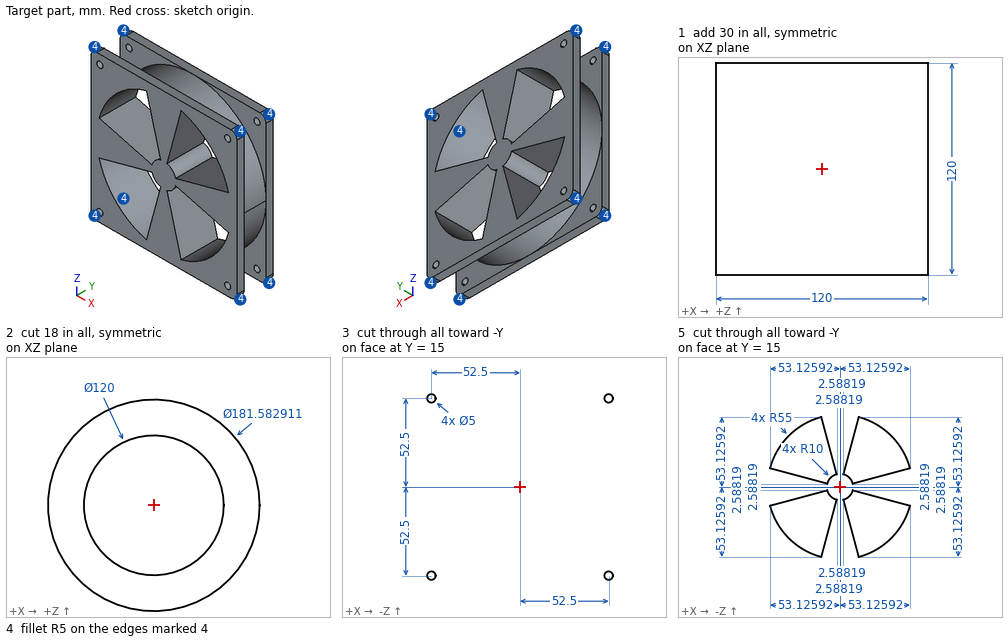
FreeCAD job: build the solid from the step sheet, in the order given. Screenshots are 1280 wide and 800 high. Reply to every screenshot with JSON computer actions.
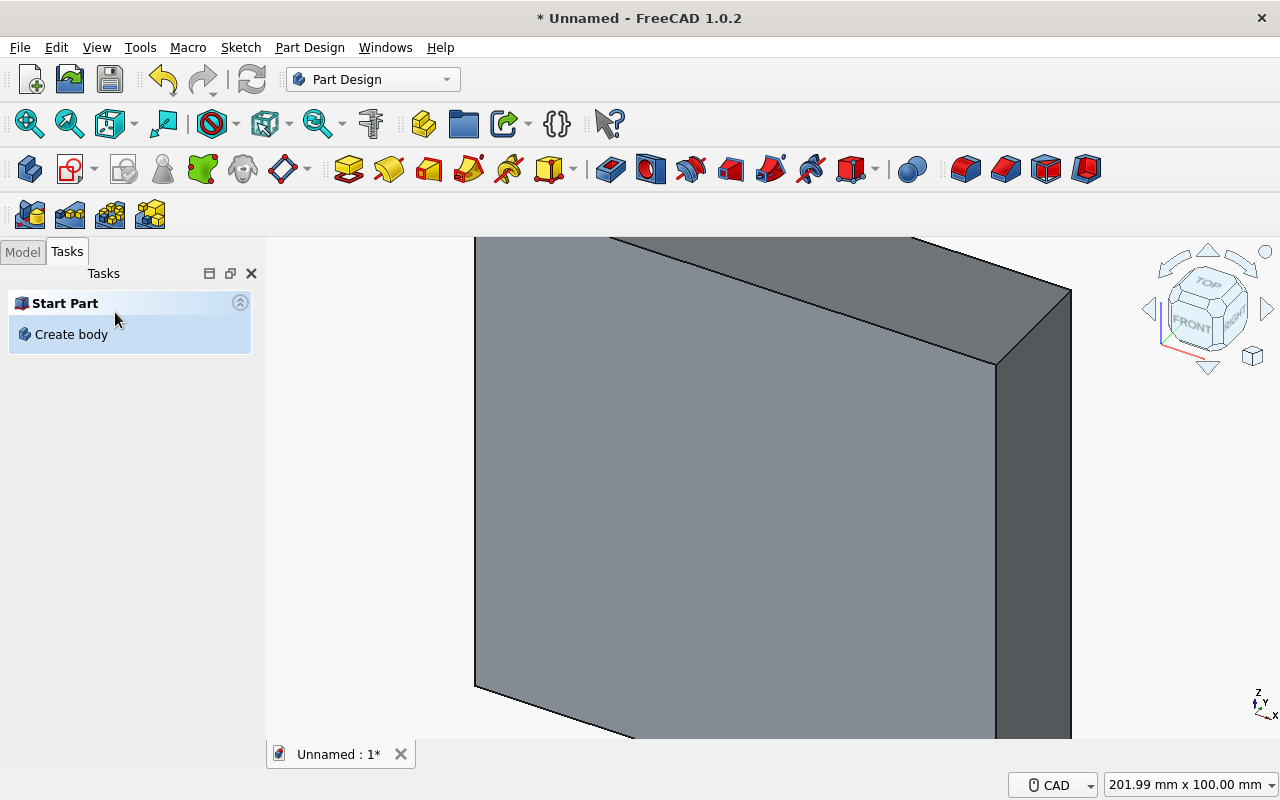
{"action": "left_click", "coordinate": [30, 124]}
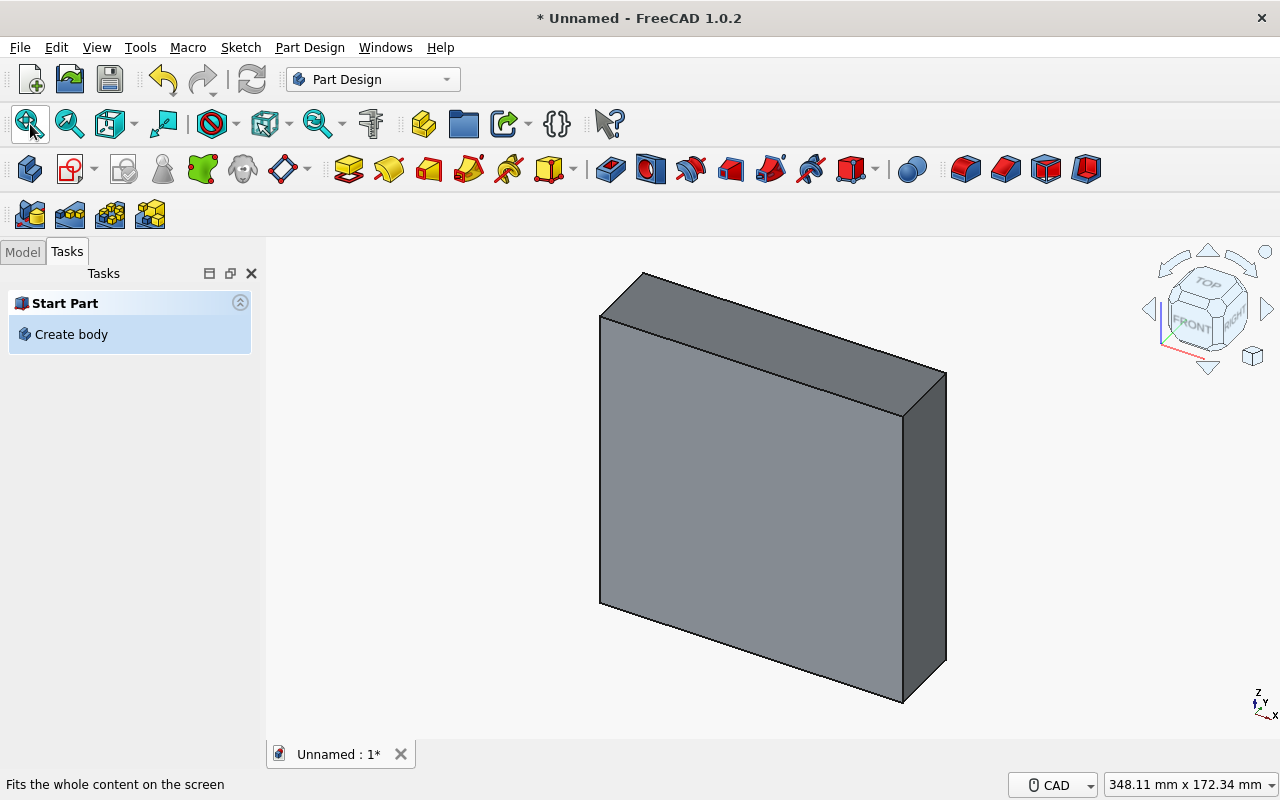
{"action": "left_click", "coordinate": [70, 170]}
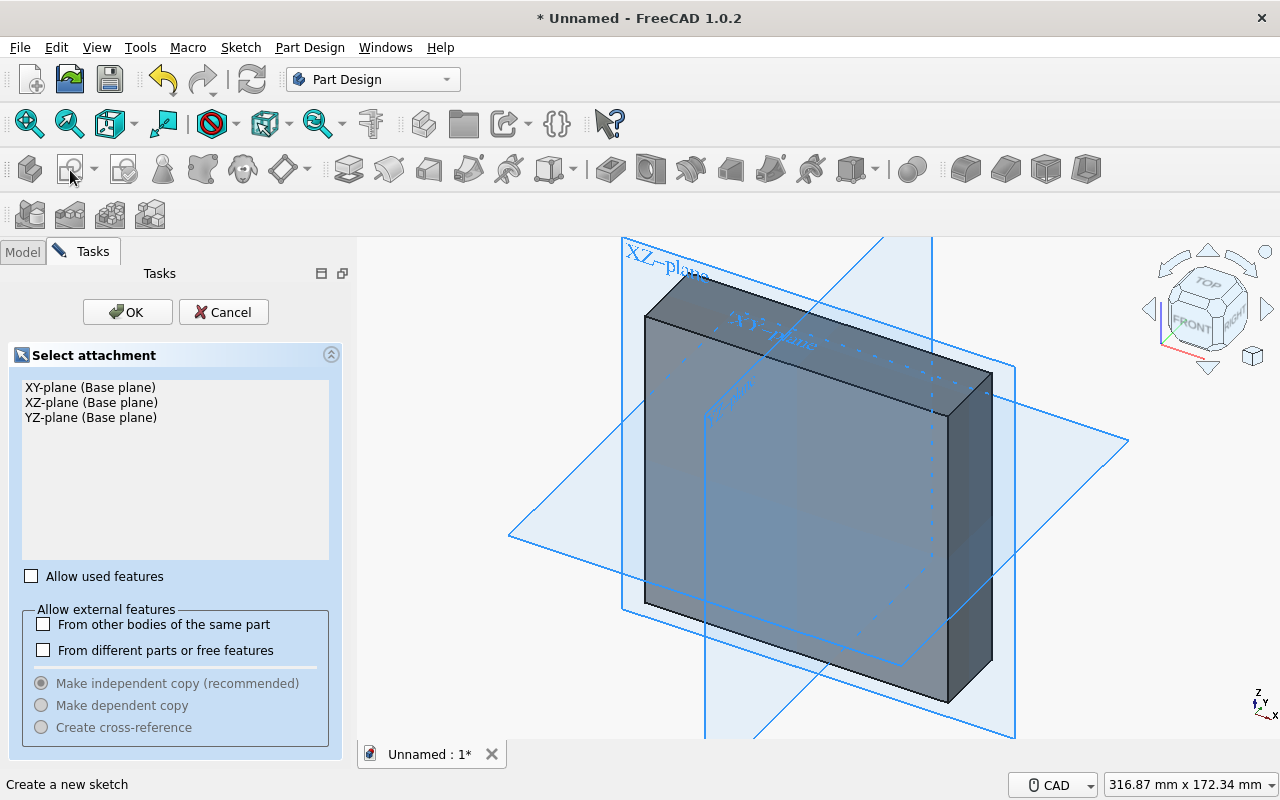
{"action": "left_click", "coordinate": [82, 402]}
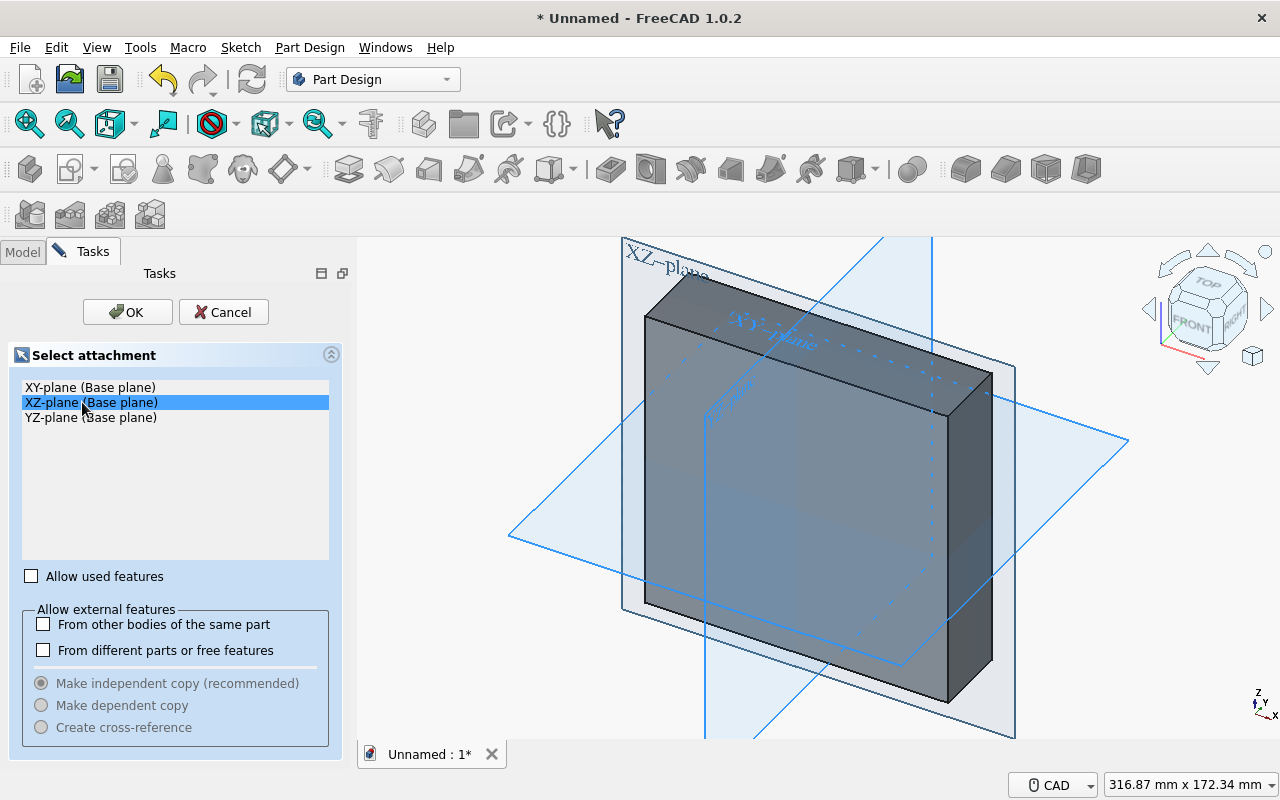
{"action": "left_click", "coordinate": [128, 312]}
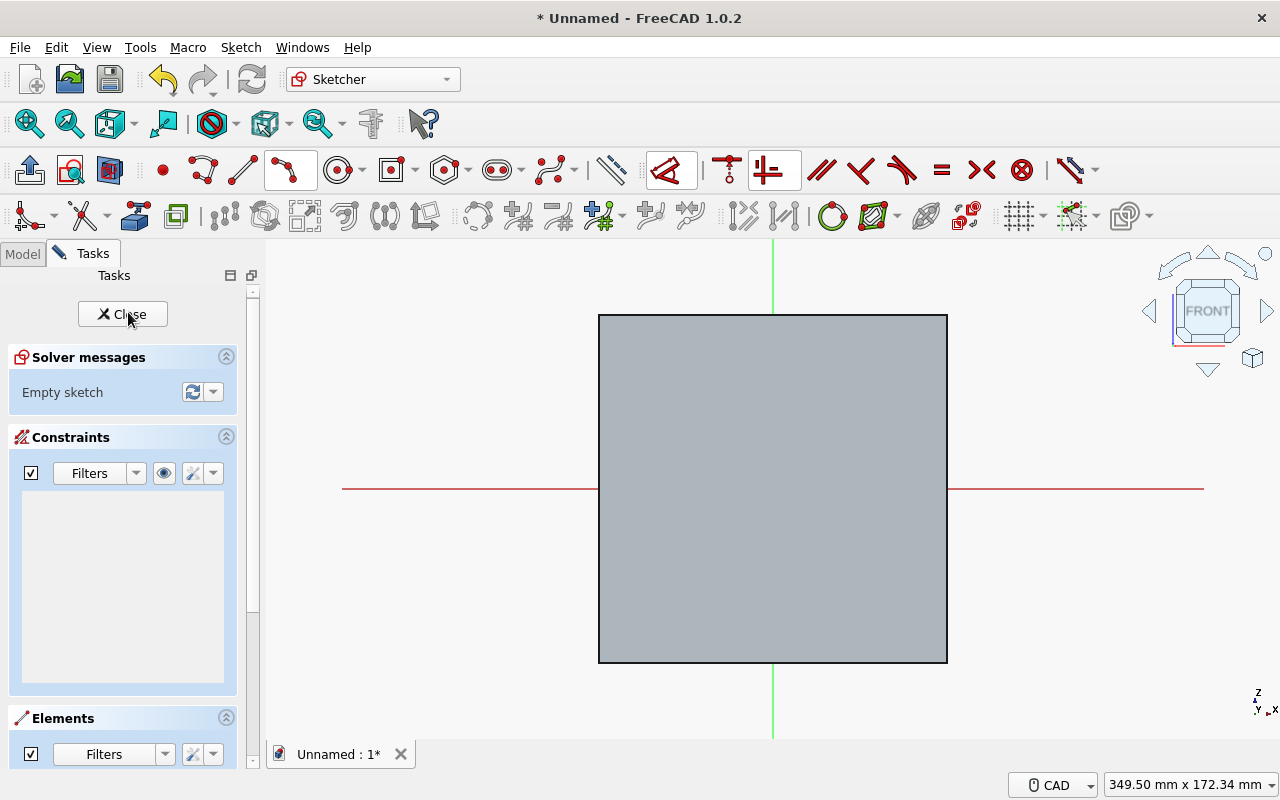
{"action": "left_click", "coordinate": [110, 170]}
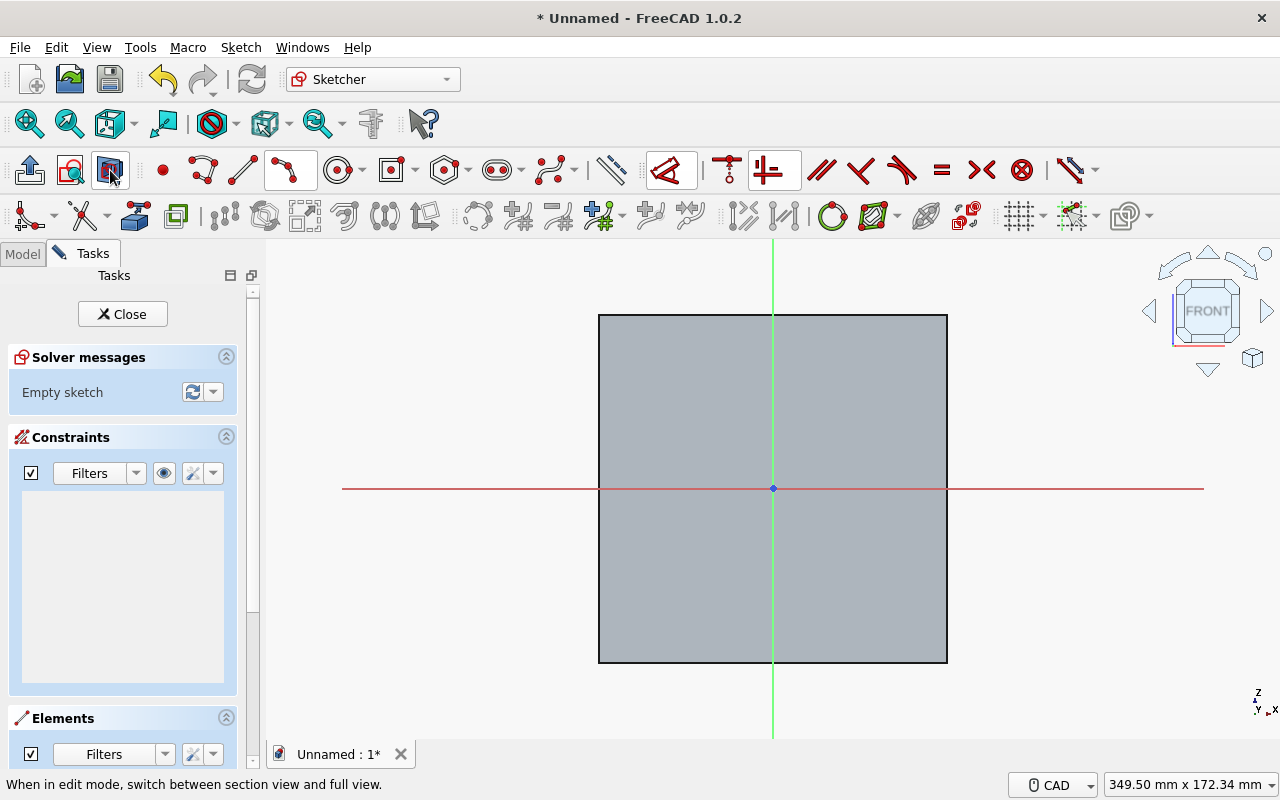
{"action": "scroll", "coordinate": [621, 489], "scroll_direction": "down", "scroll_amount": 3}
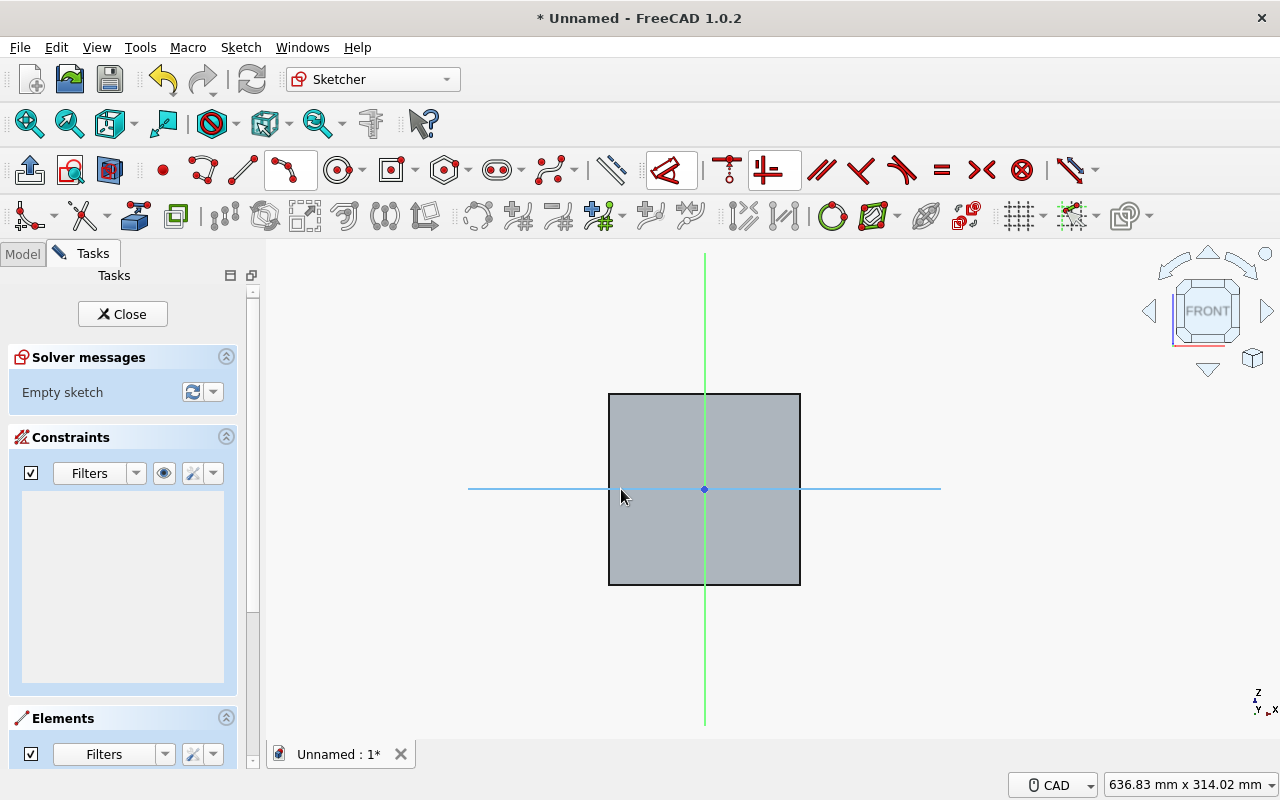
{"action": "left_click", "coordinate": [338, 170]}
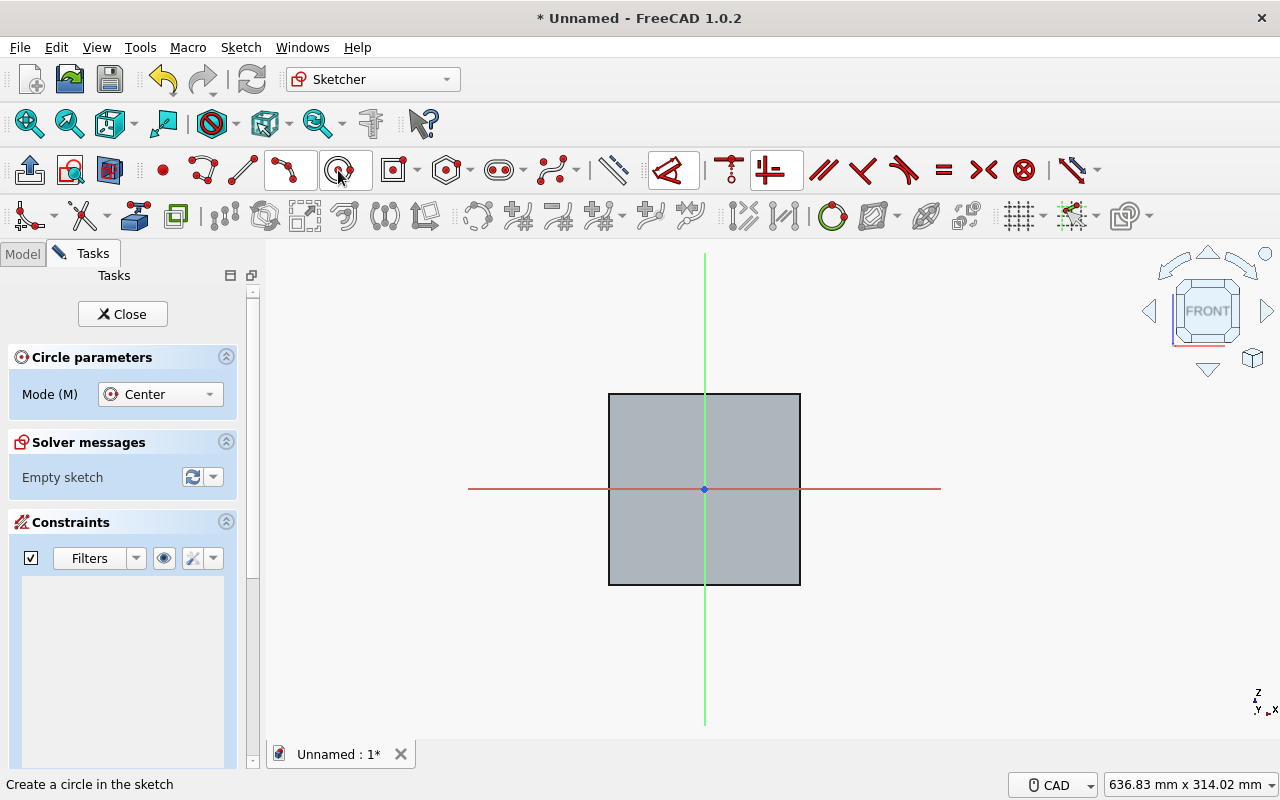
{"action": "left_click", "coordinate": [705, 489]}
{"action": "left_click", "coordinate": [807, 387]}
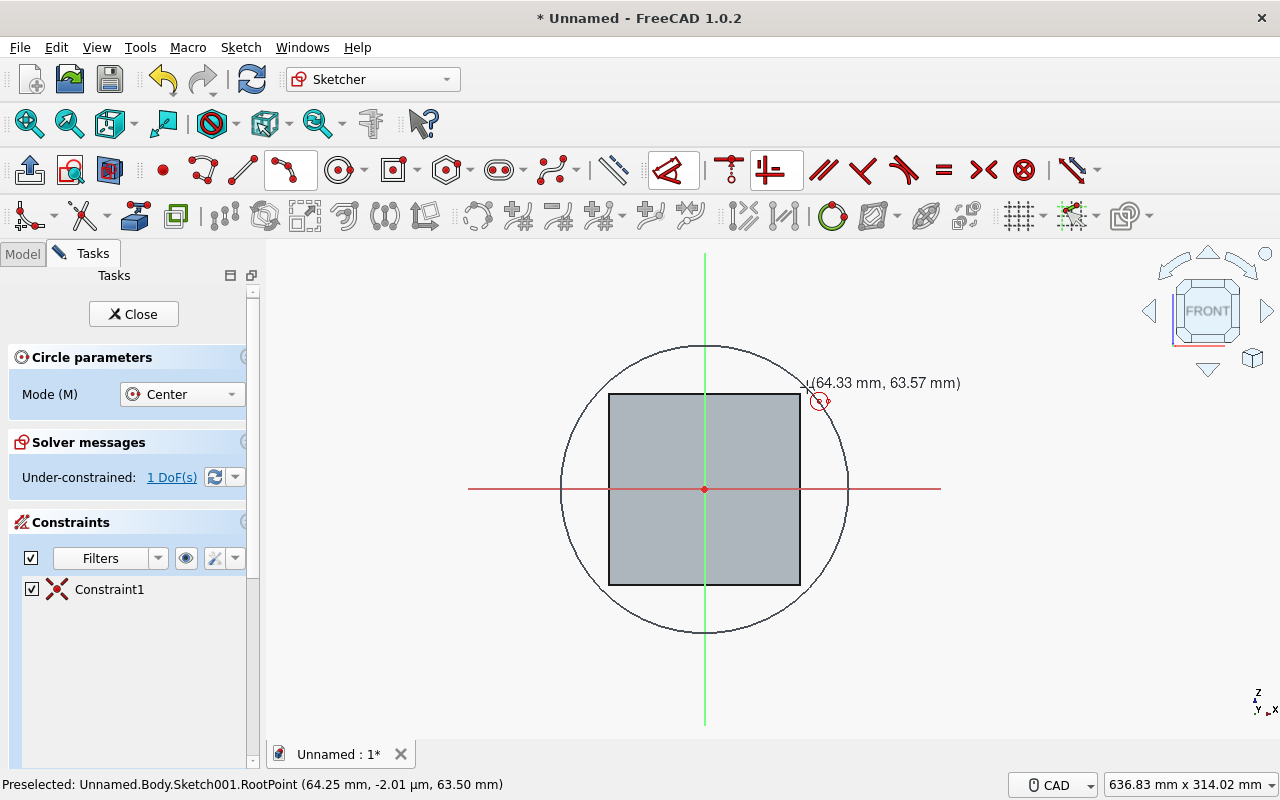
{"action": "left_click", "coordinate": [705, 489]}
{"action": "left_click", "coordinate": [772, 422]}
{"action": "key", "text": "Escape"}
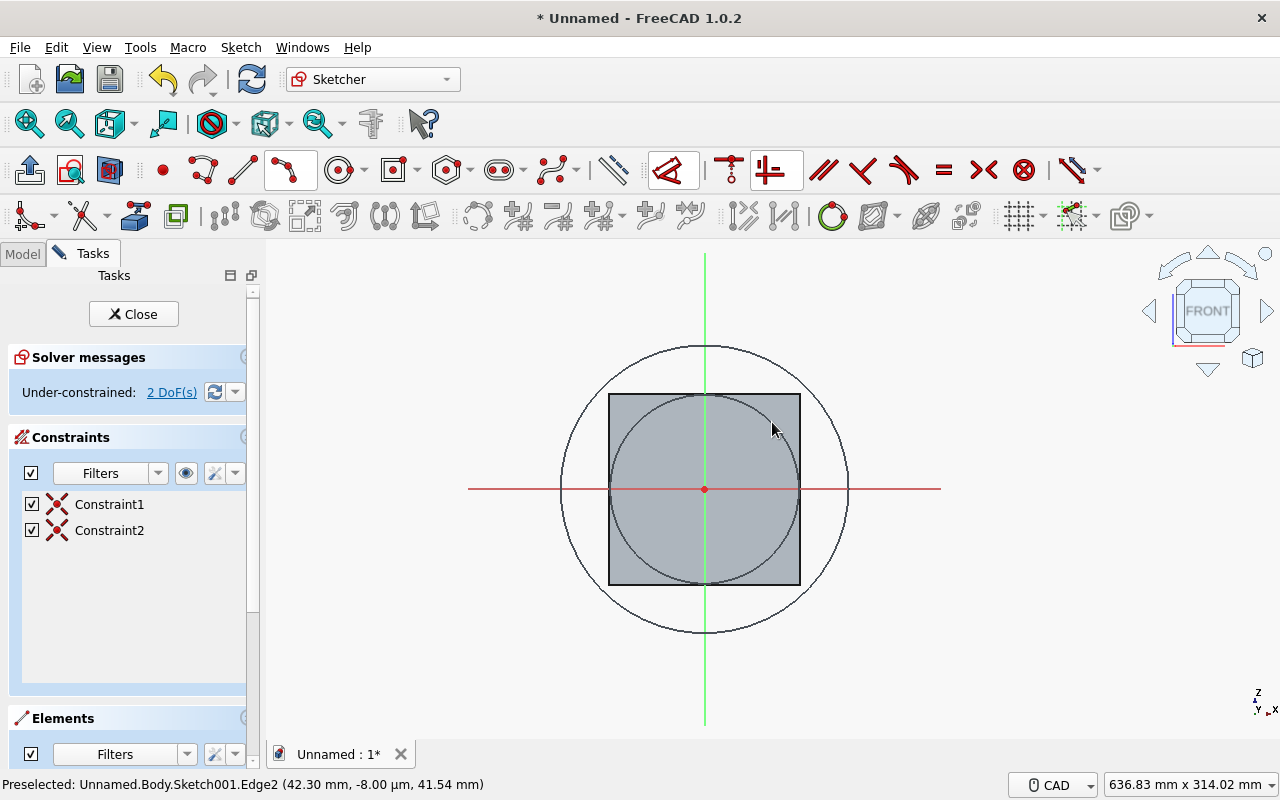
{"action": "left_click", "coordinate": [806, 387]}